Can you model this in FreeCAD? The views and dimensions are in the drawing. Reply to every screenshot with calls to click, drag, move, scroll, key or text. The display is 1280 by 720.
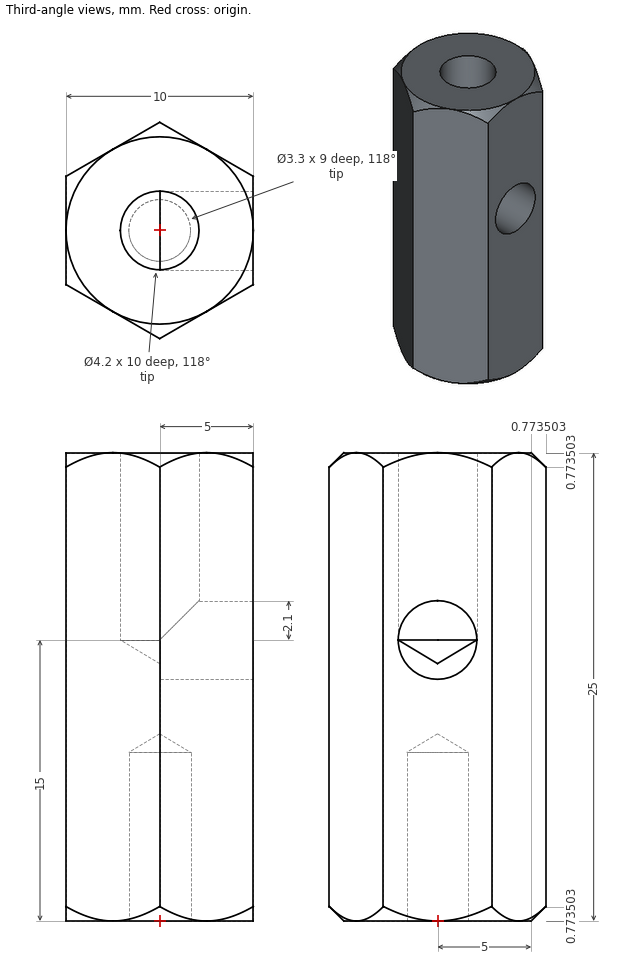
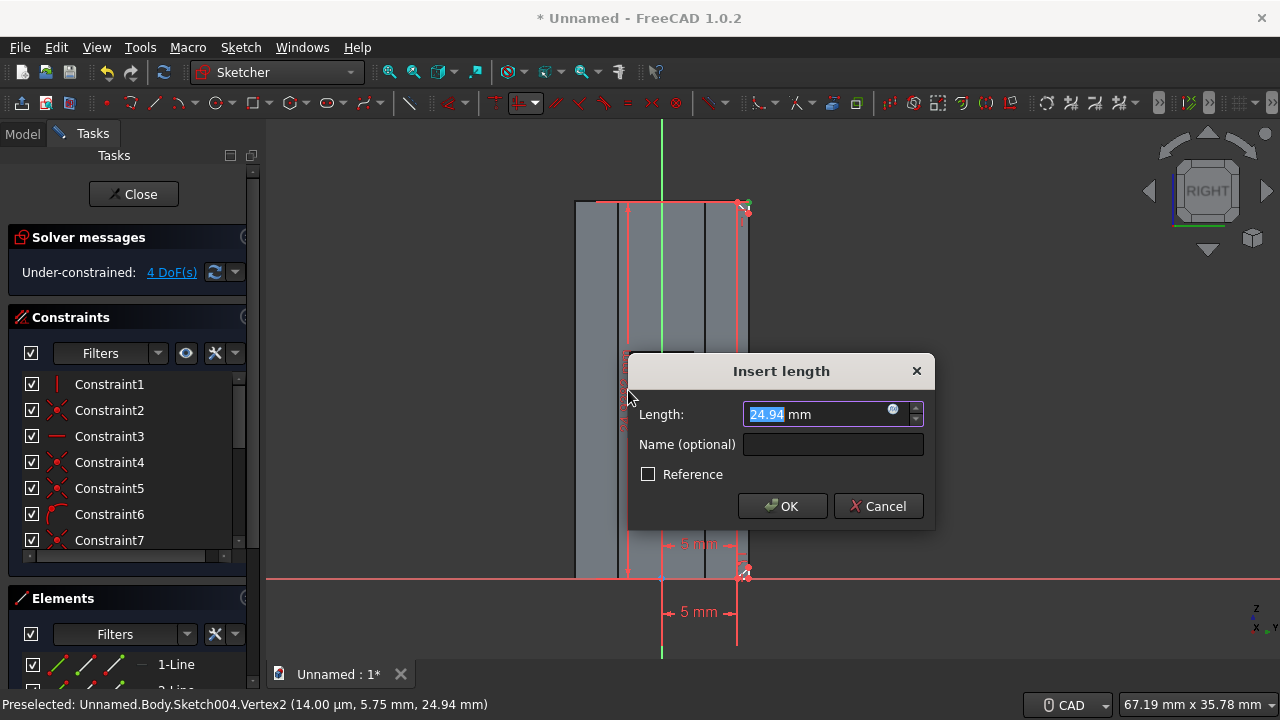
text(25)
key(Return)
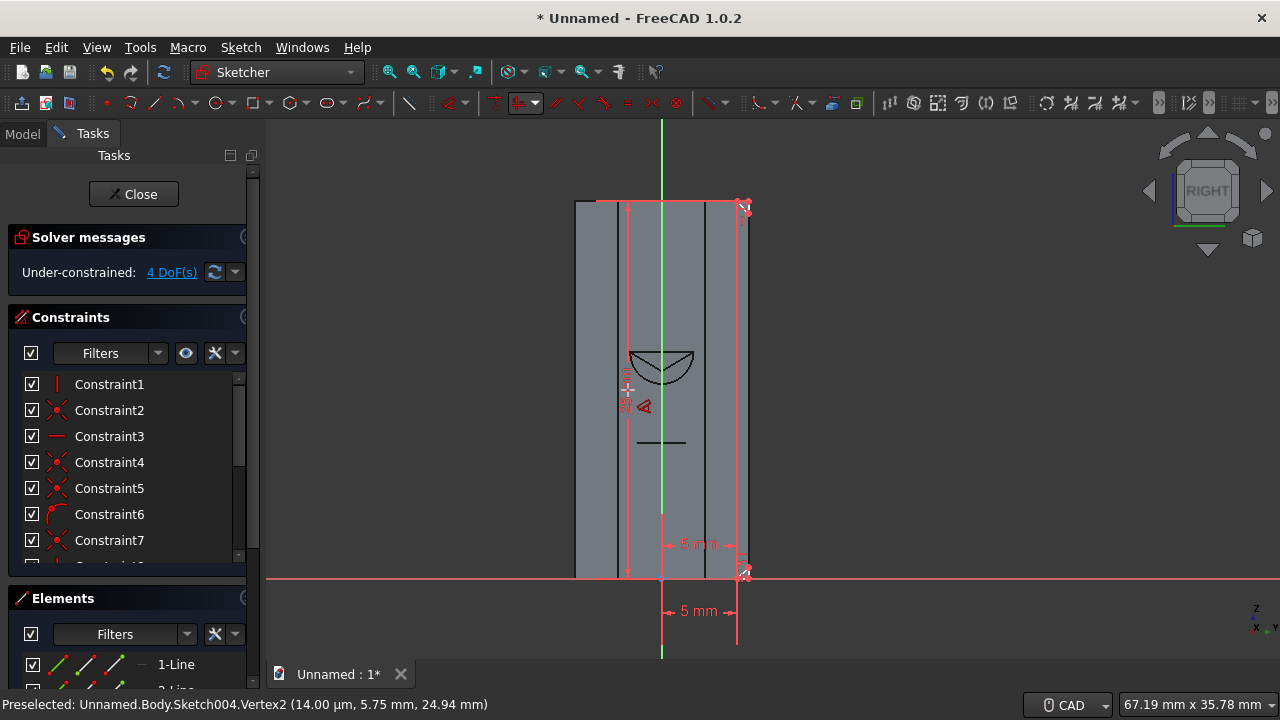
scroll(749, 206, up, 7)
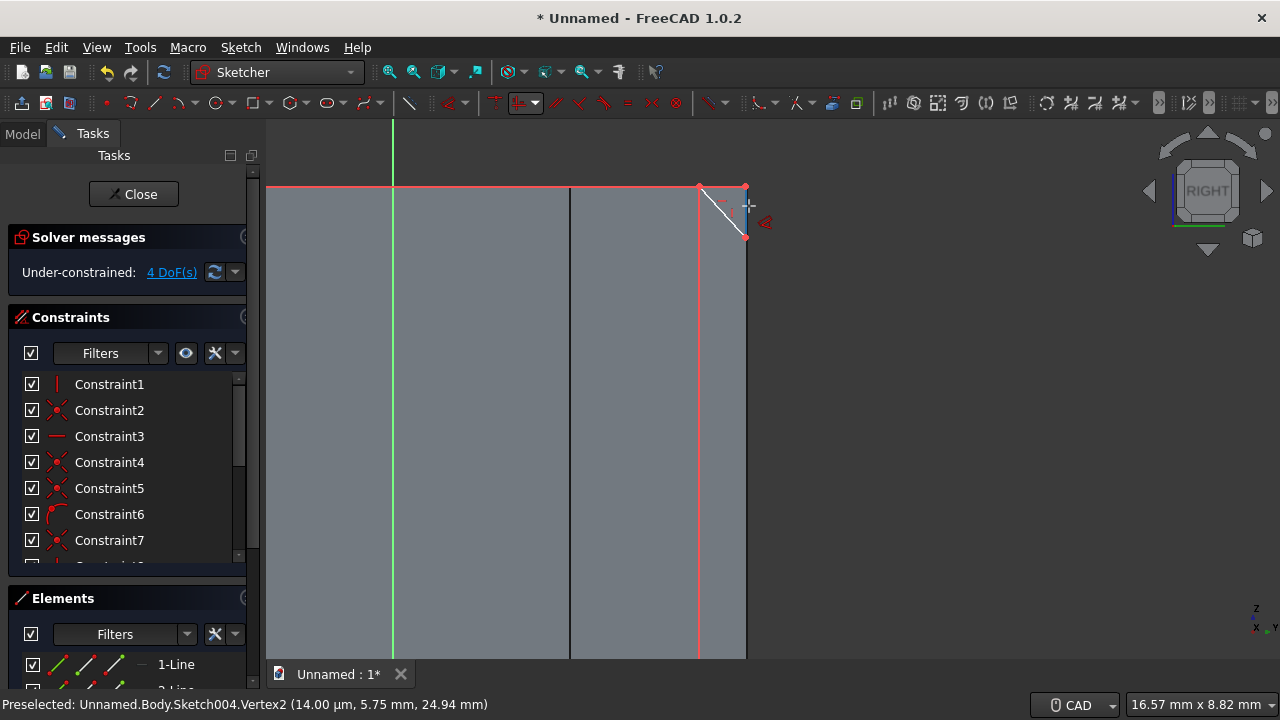
click(746, 207)
click(780, 212)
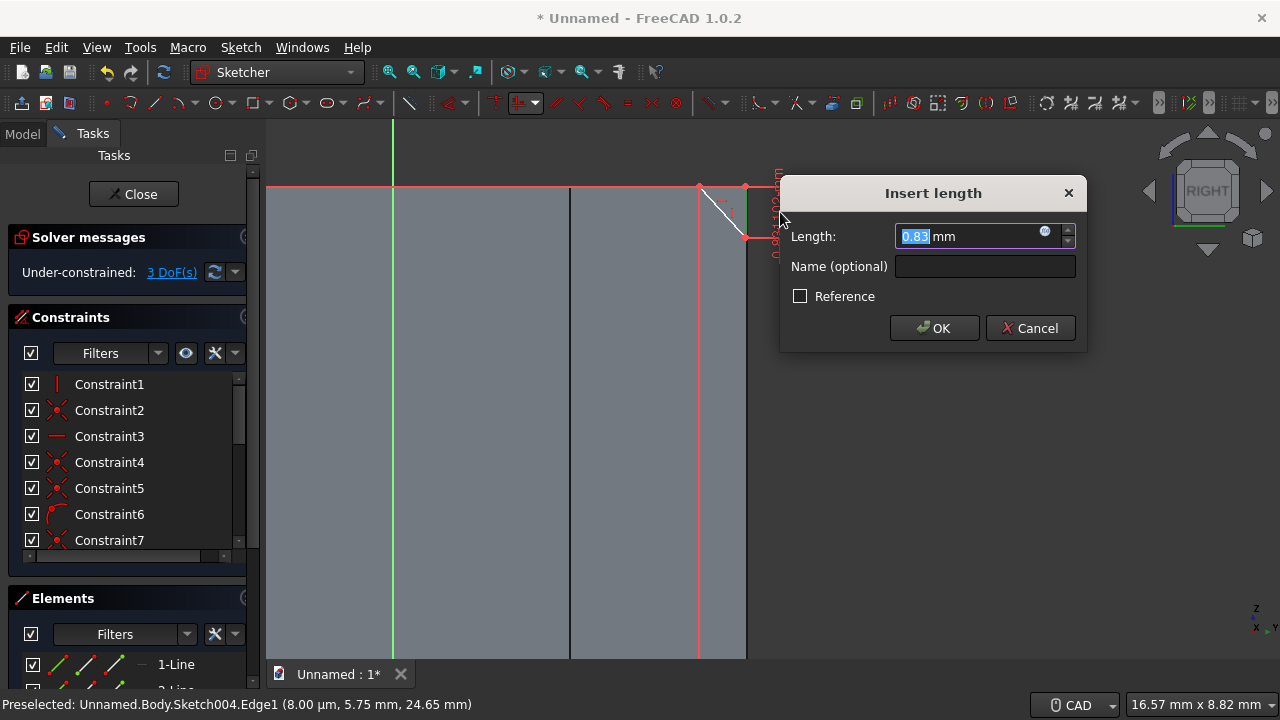
text(0.773503)
key(Return)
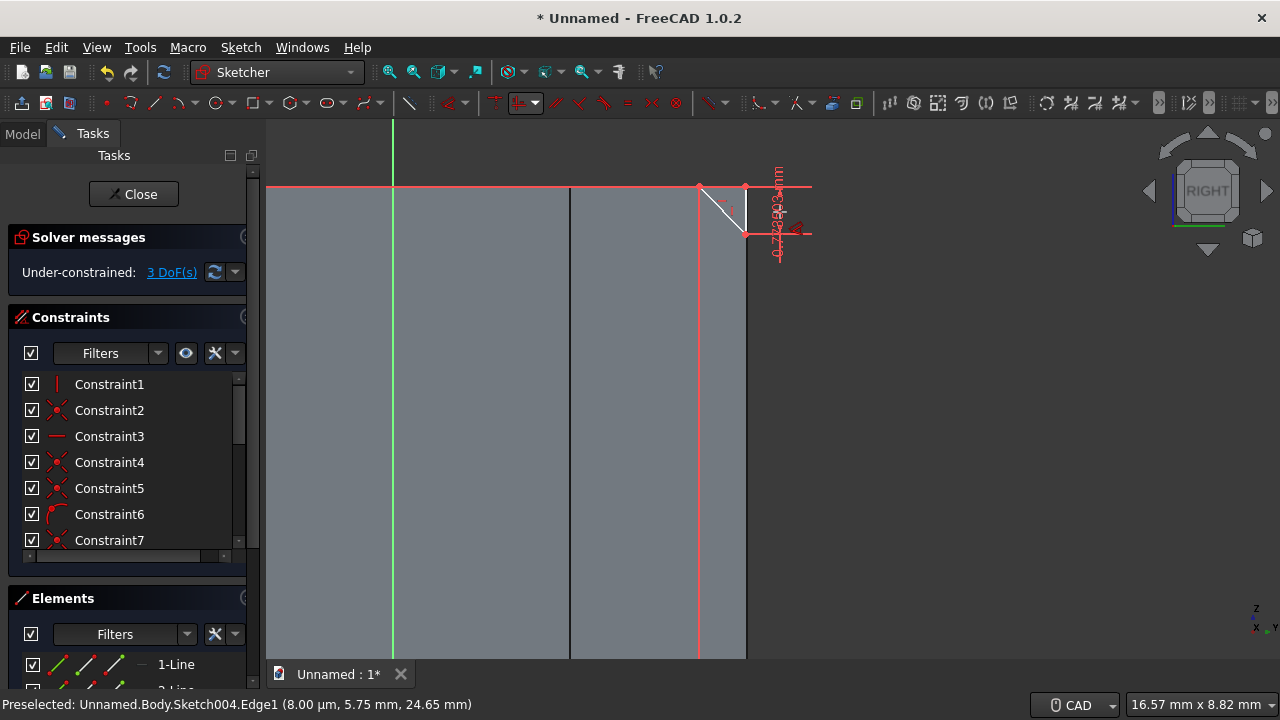
click(732, 187)
click(723, 153)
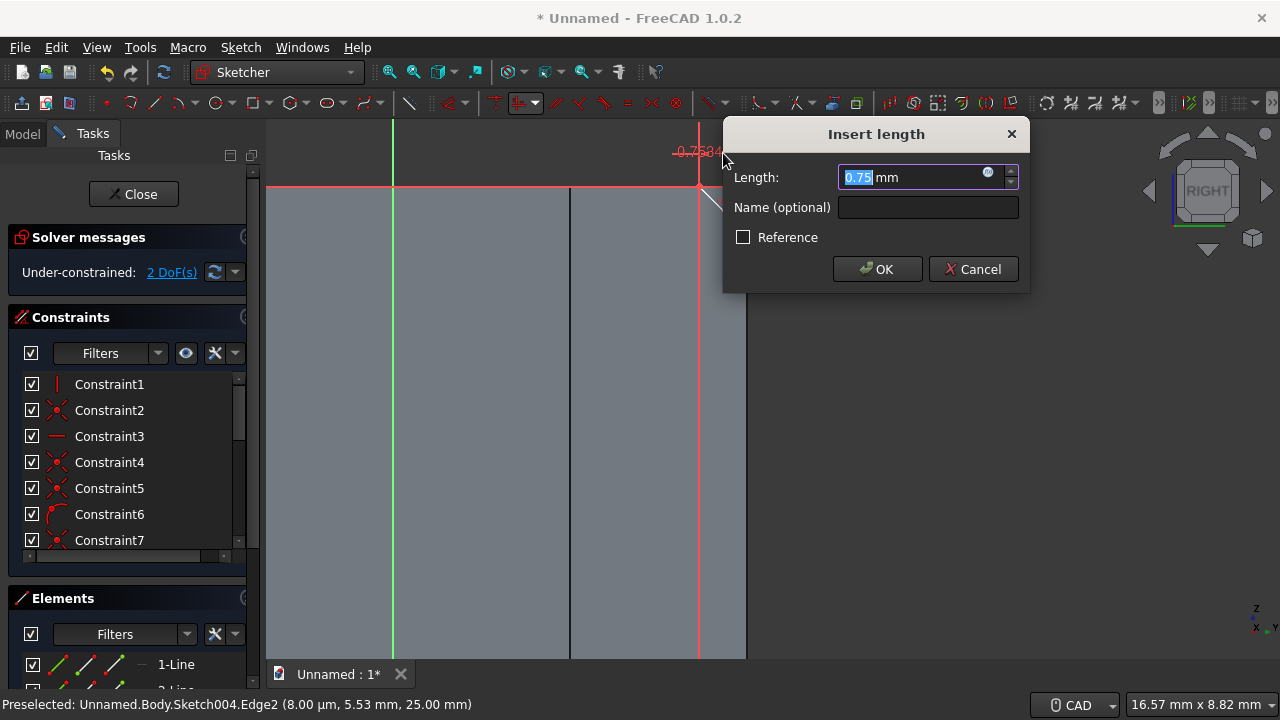
text(0.773503)
key(Return)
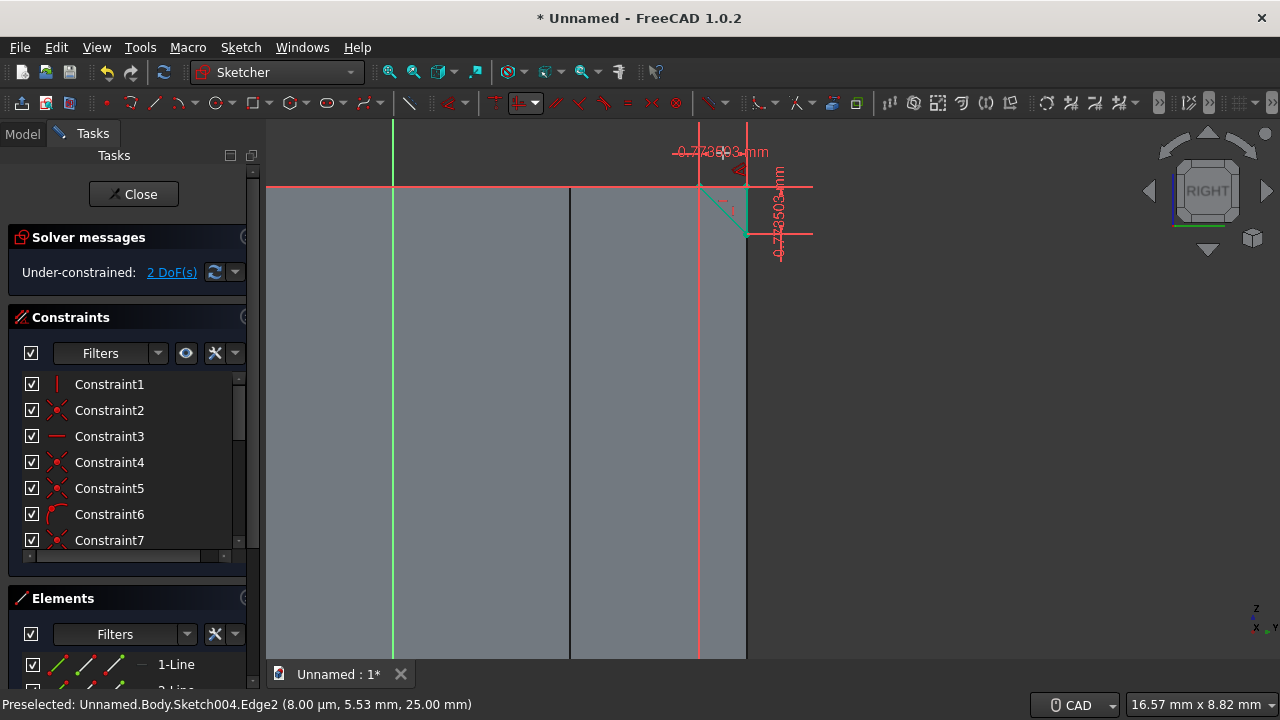
scroll(748, 205, down, 7)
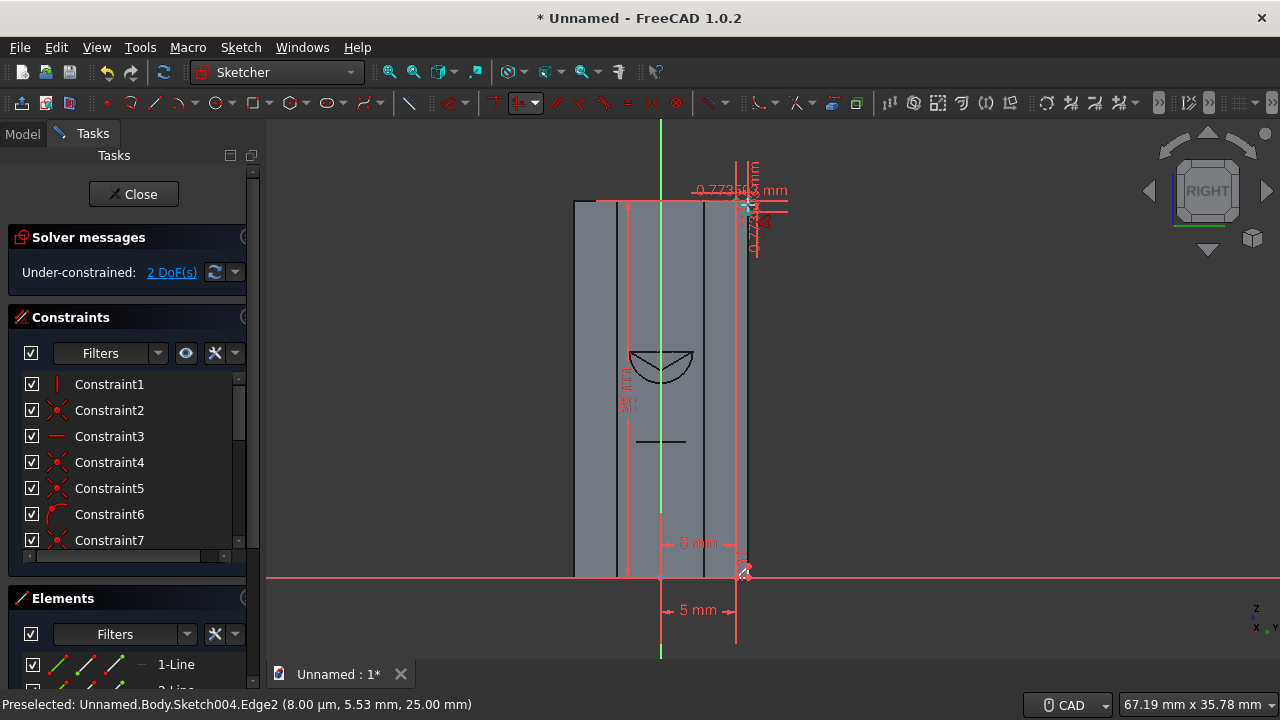
scroll(740, 578, up, 9)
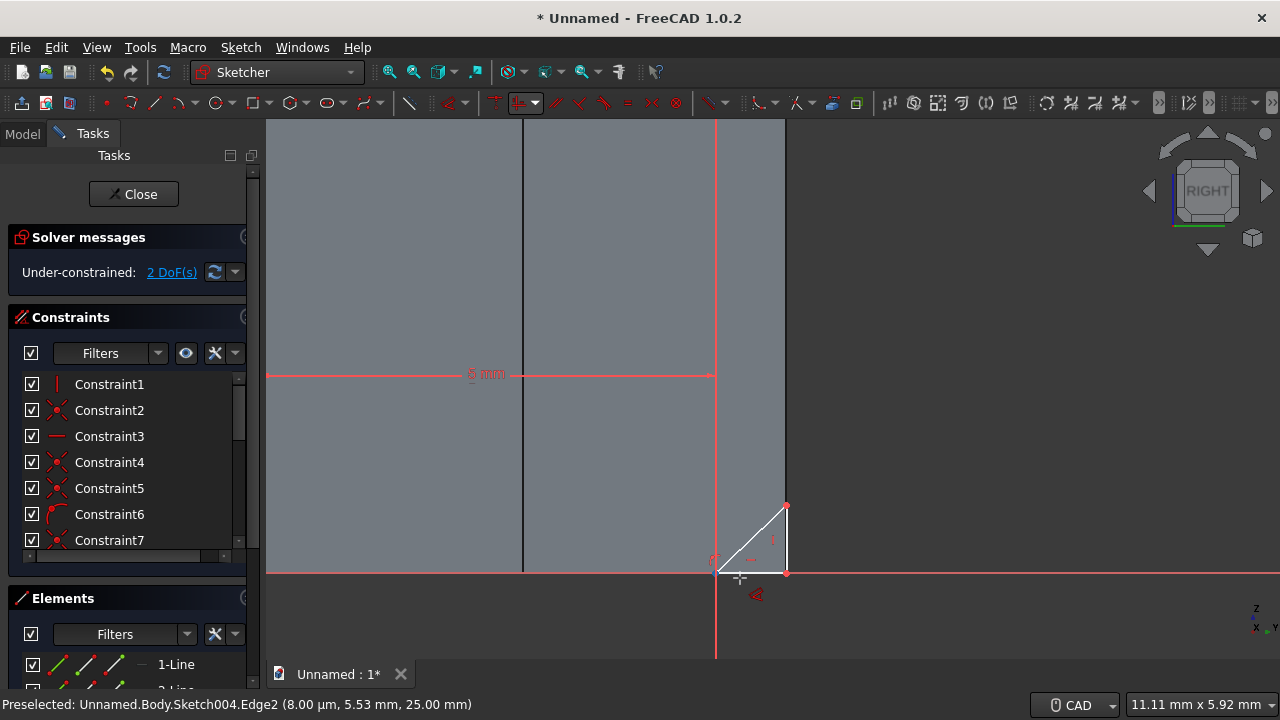
click(737, 573)
click(751, 607)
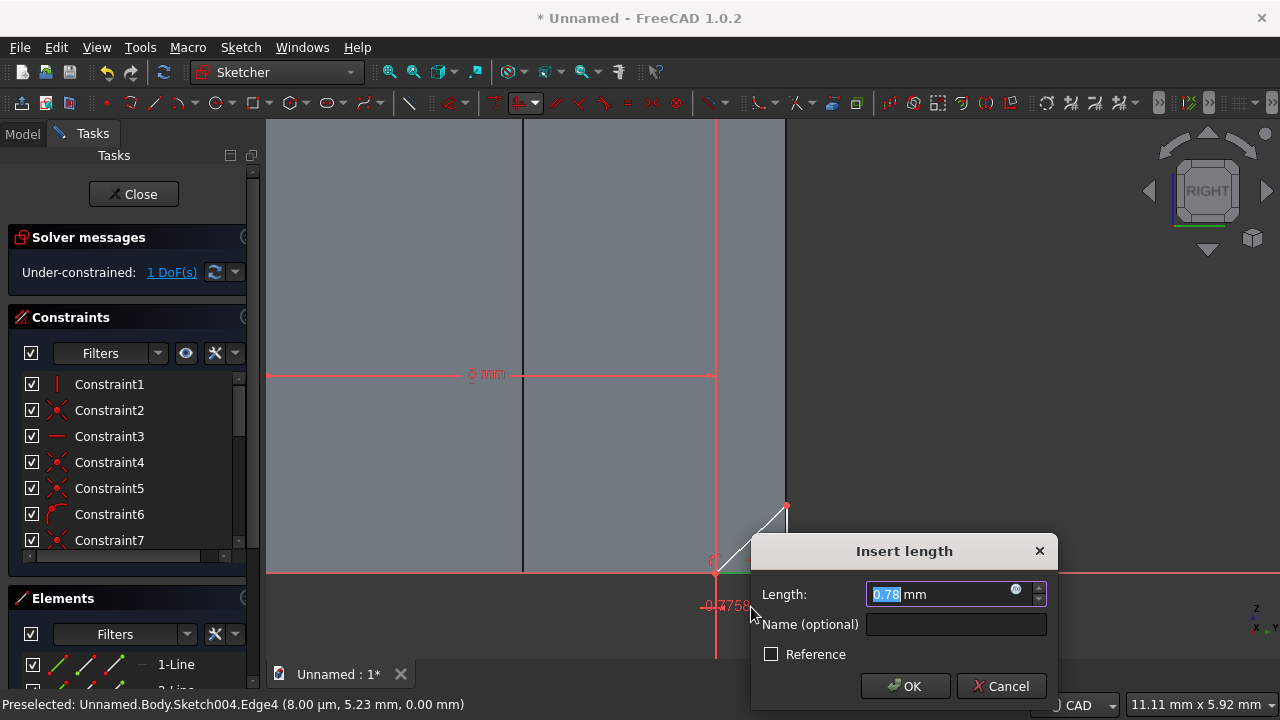
text(0.773503)
key(Return)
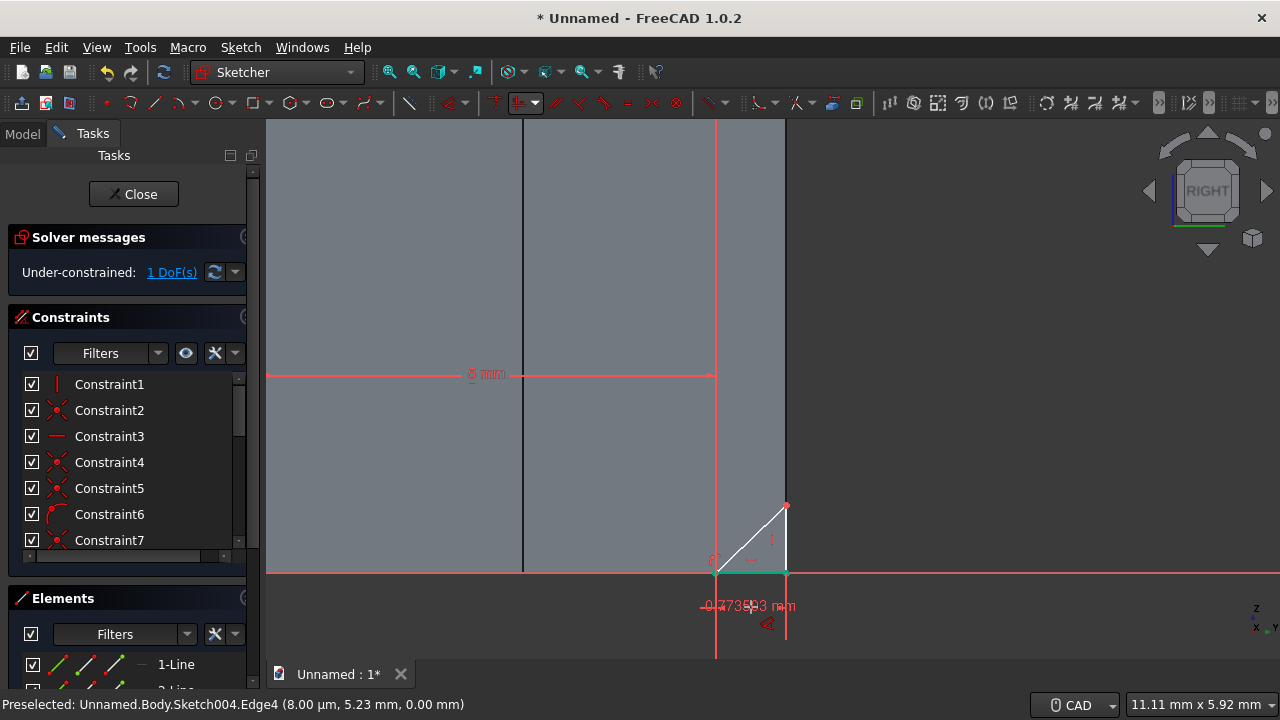
click(786, 553)
click(820, 539)